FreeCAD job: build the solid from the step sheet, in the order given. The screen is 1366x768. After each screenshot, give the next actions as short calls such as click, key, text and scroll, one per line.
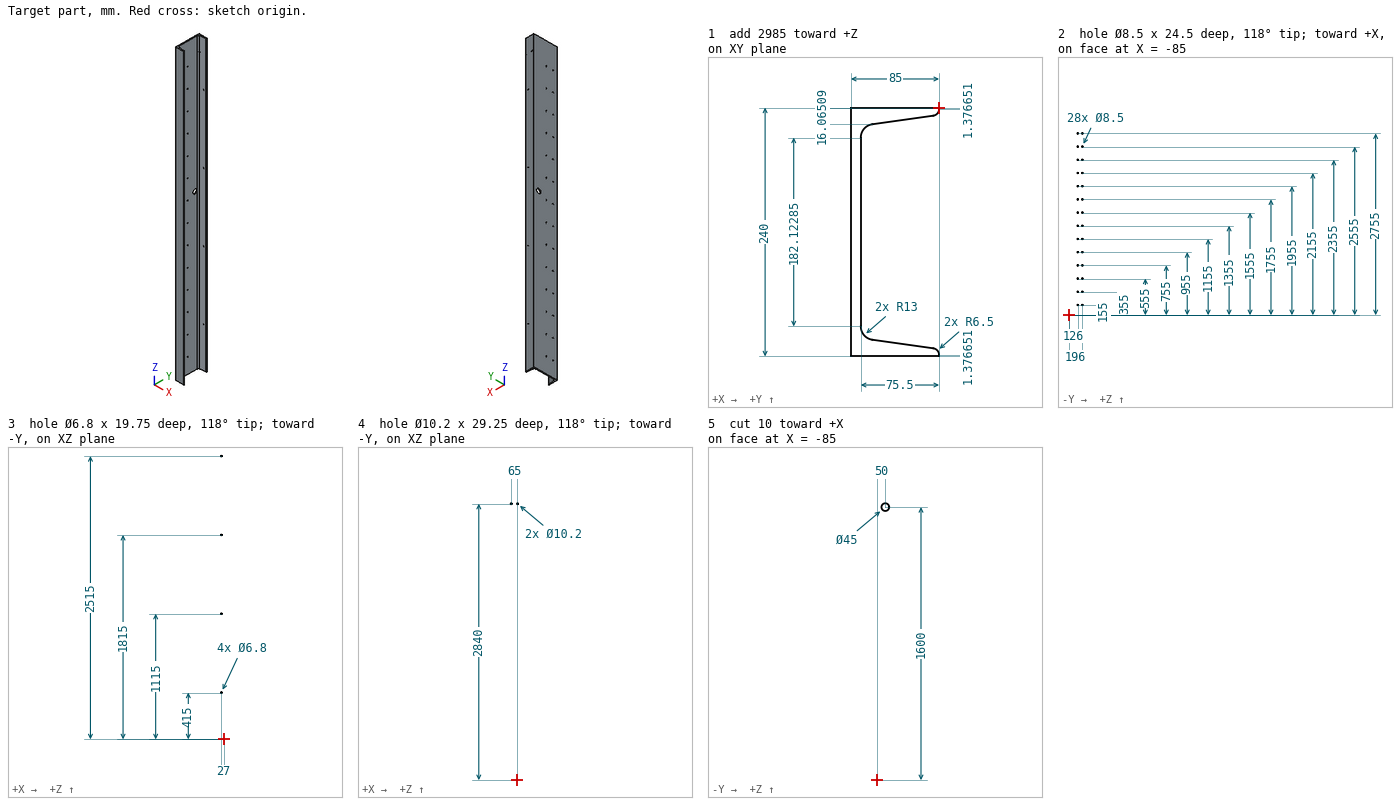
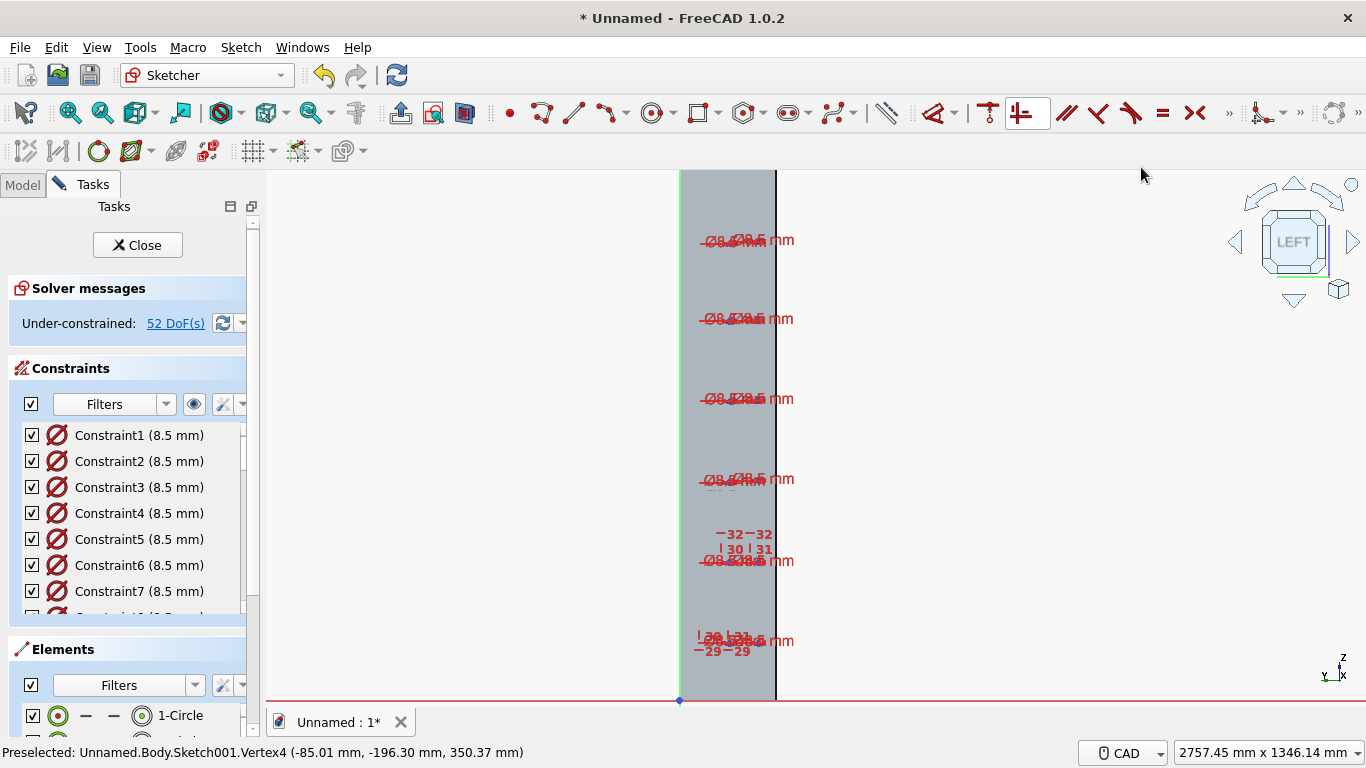
click(729, 563)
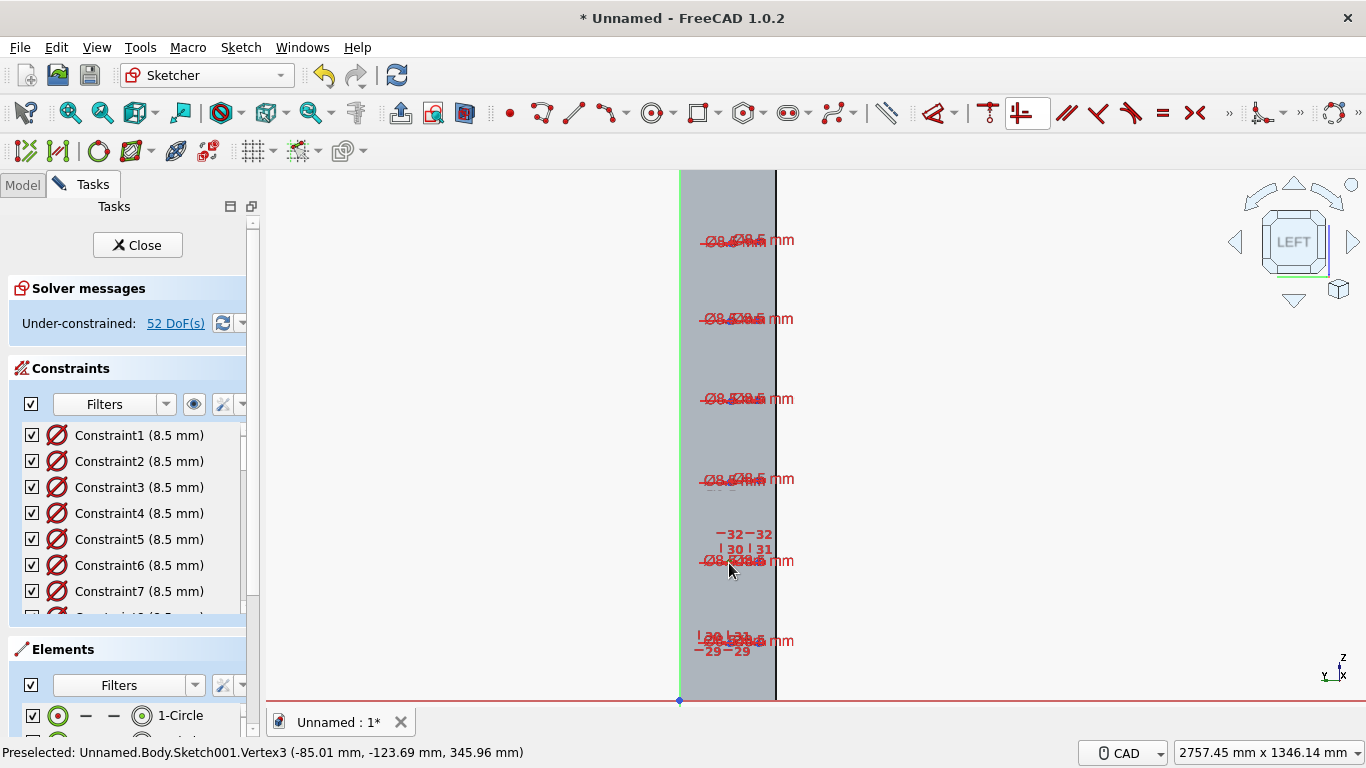
click(729, 483)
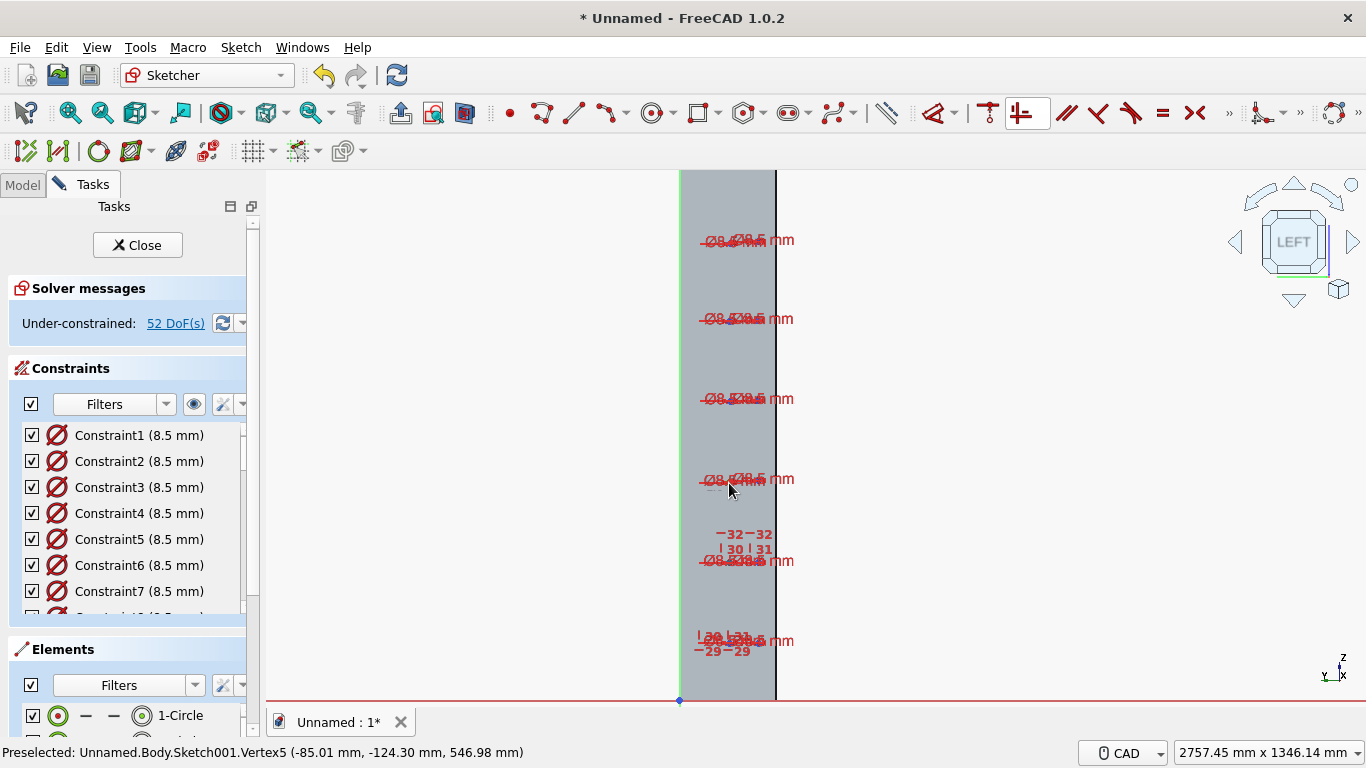
key(v)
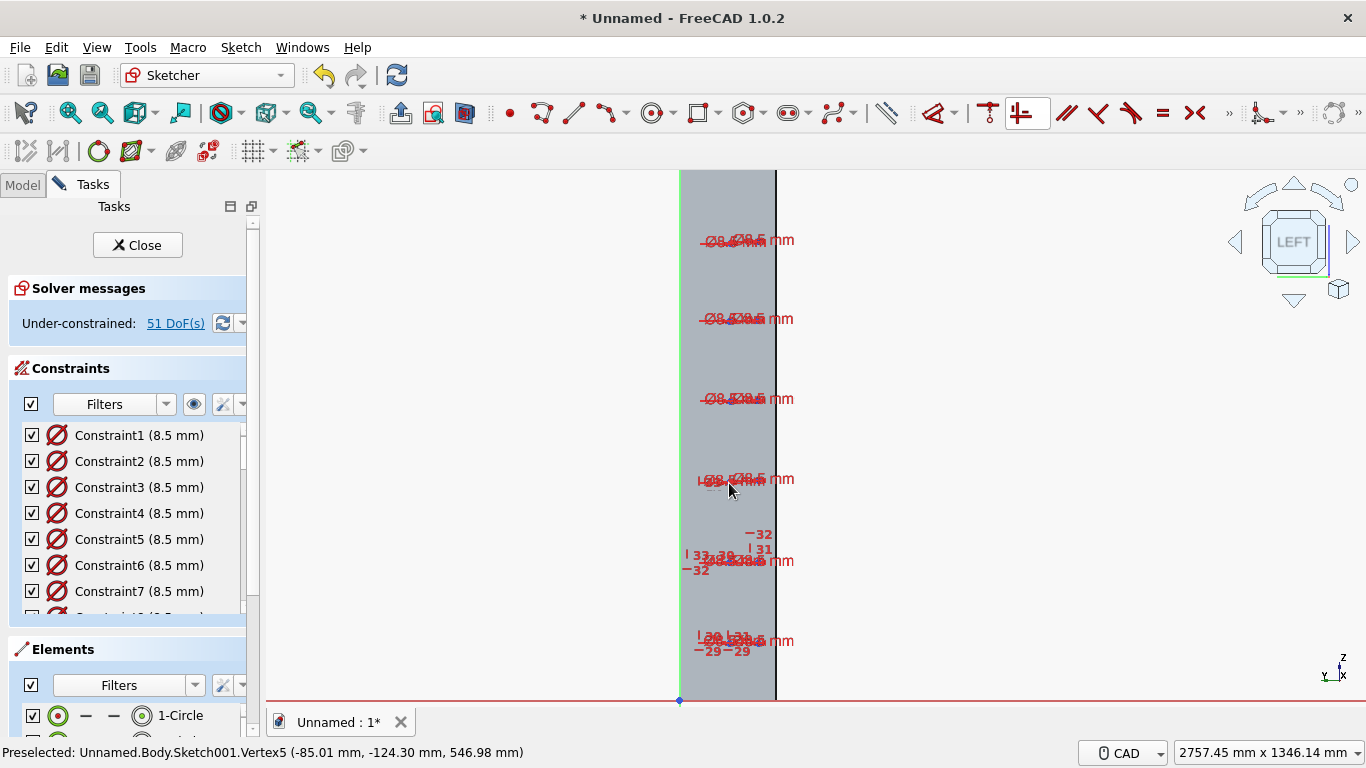
click(758, 563)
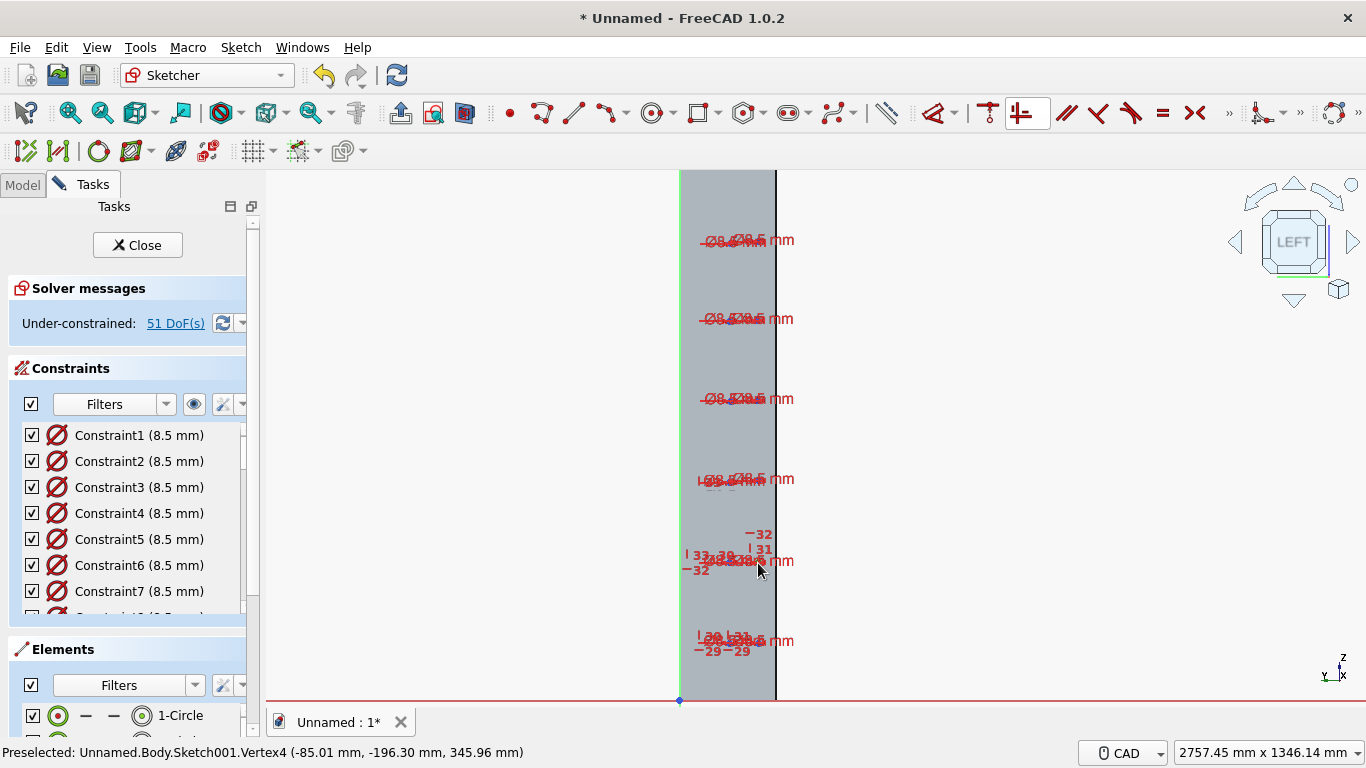
click(758, 481)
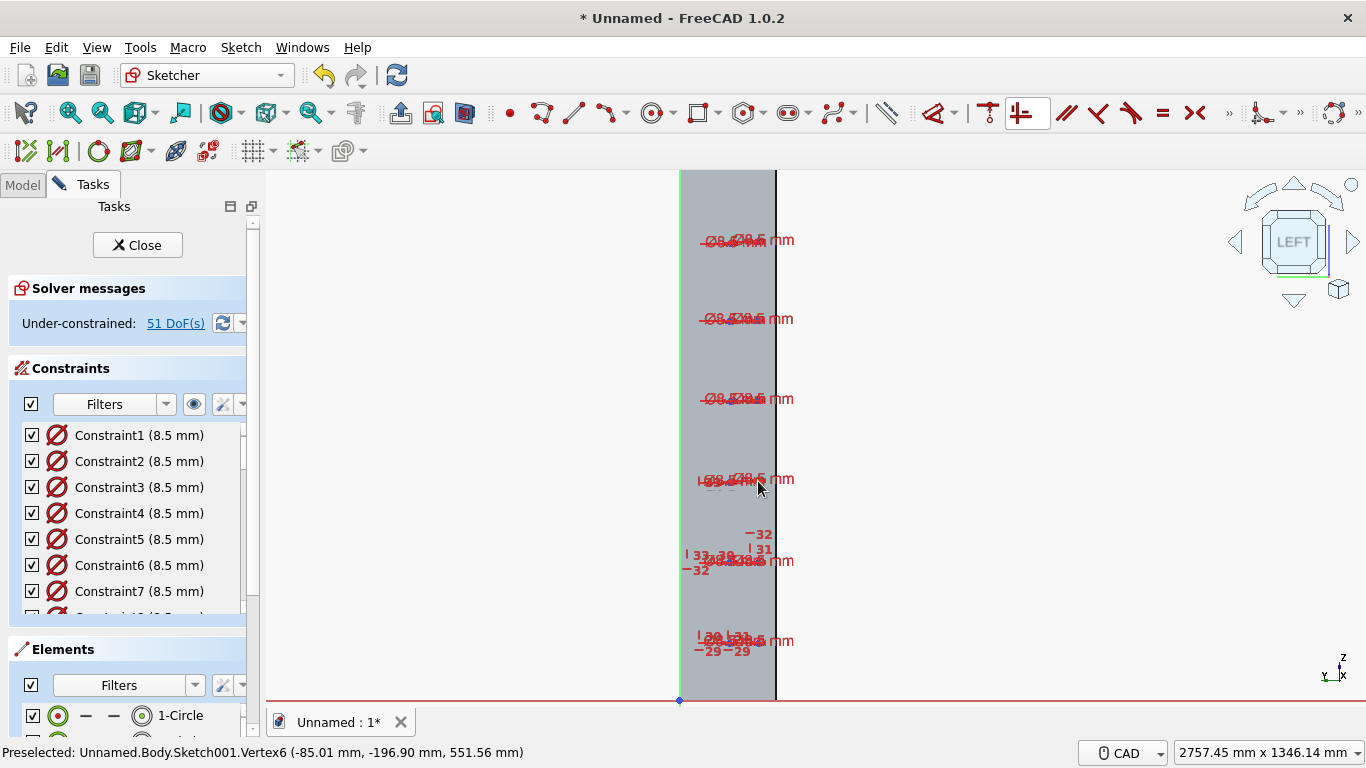
click(1044, 114)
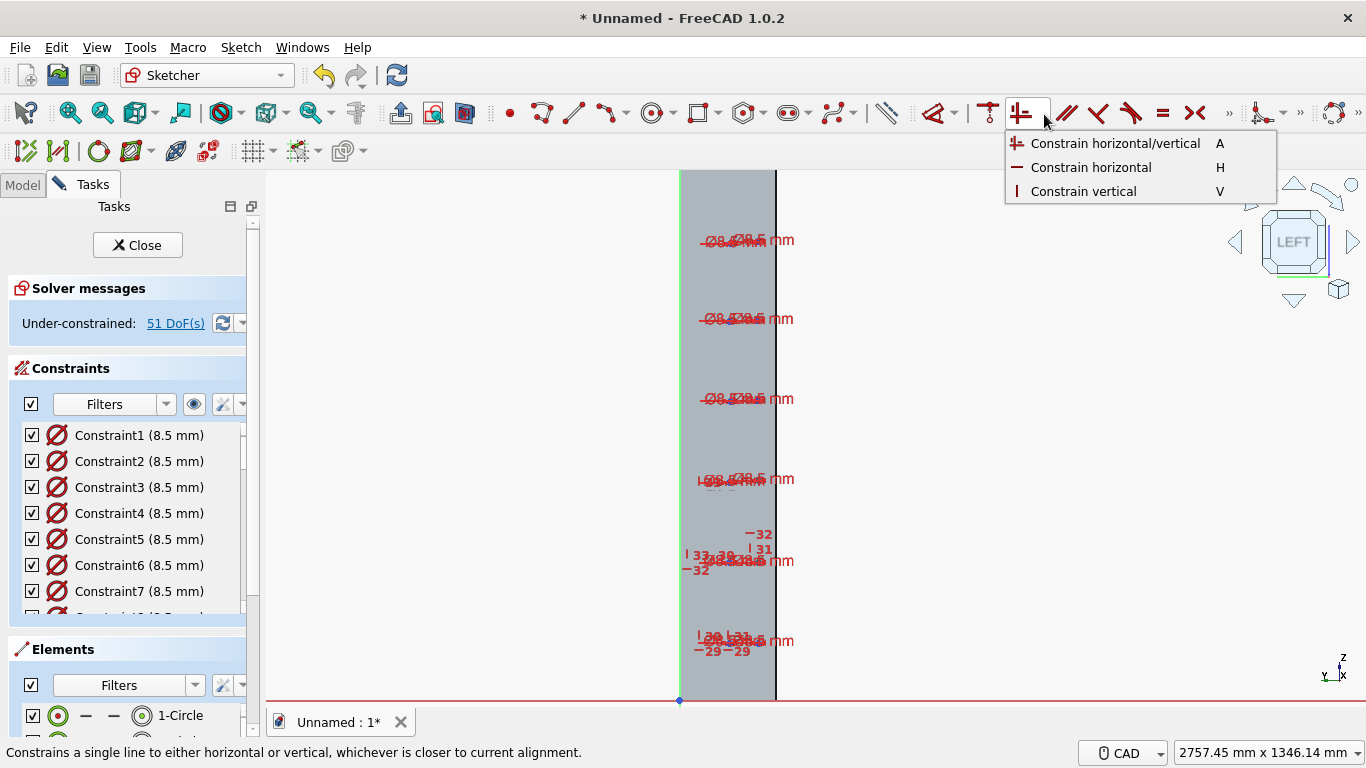
click(1141, 191)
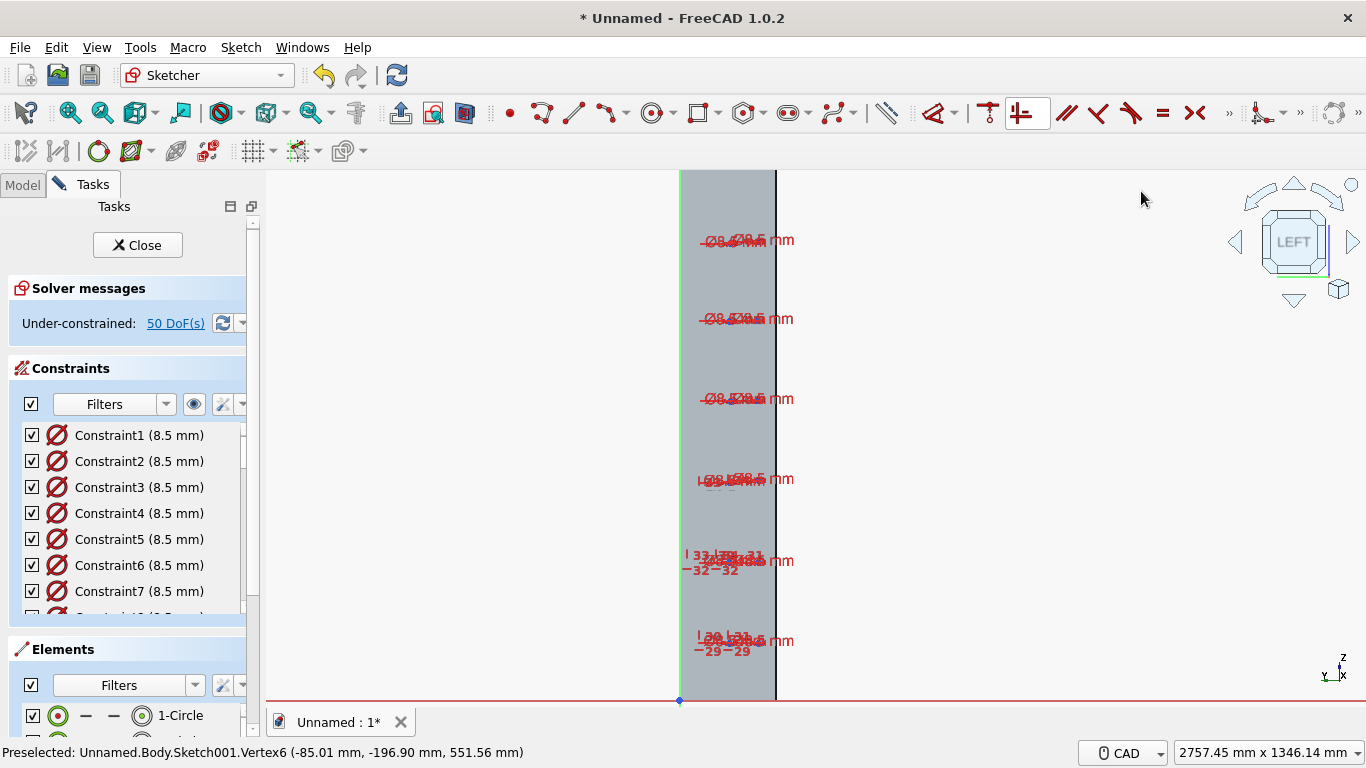
scroll(729, 483, up, 4)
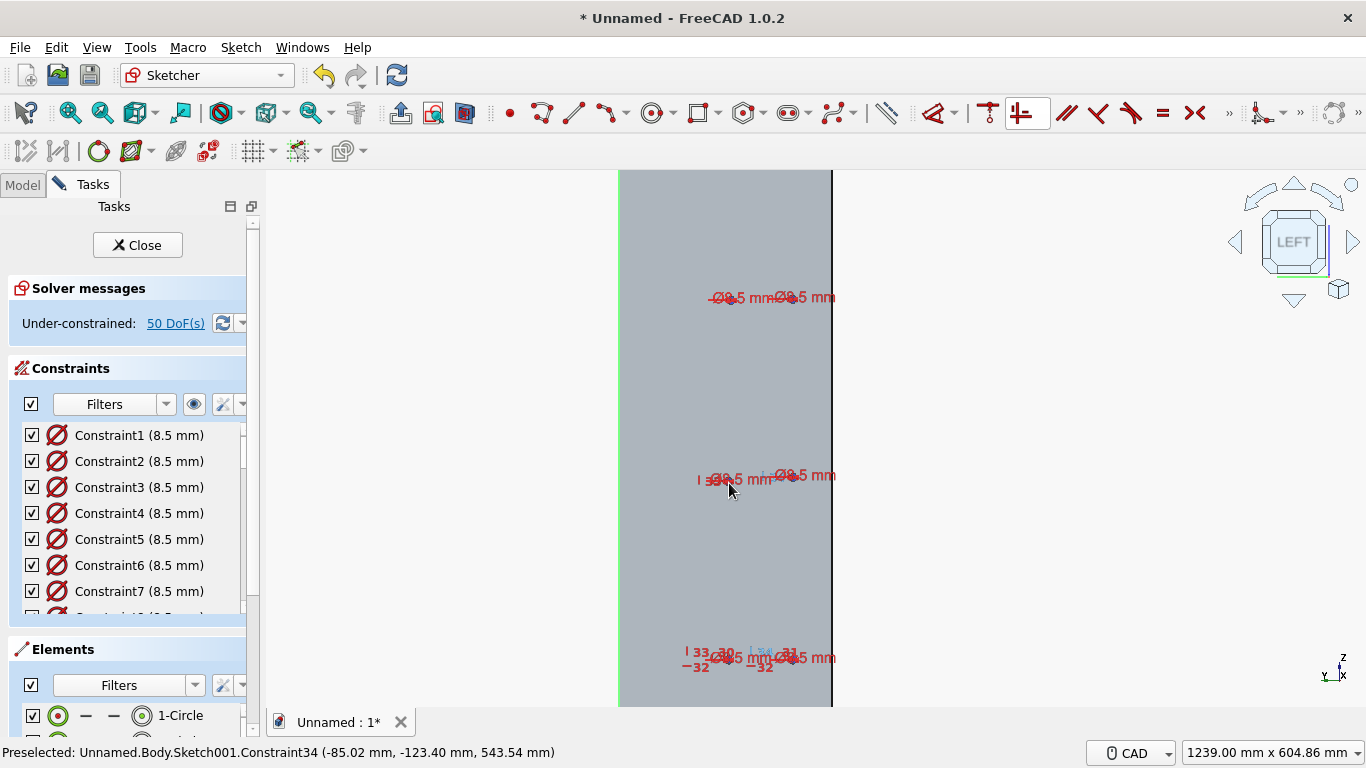
click(729, 481)